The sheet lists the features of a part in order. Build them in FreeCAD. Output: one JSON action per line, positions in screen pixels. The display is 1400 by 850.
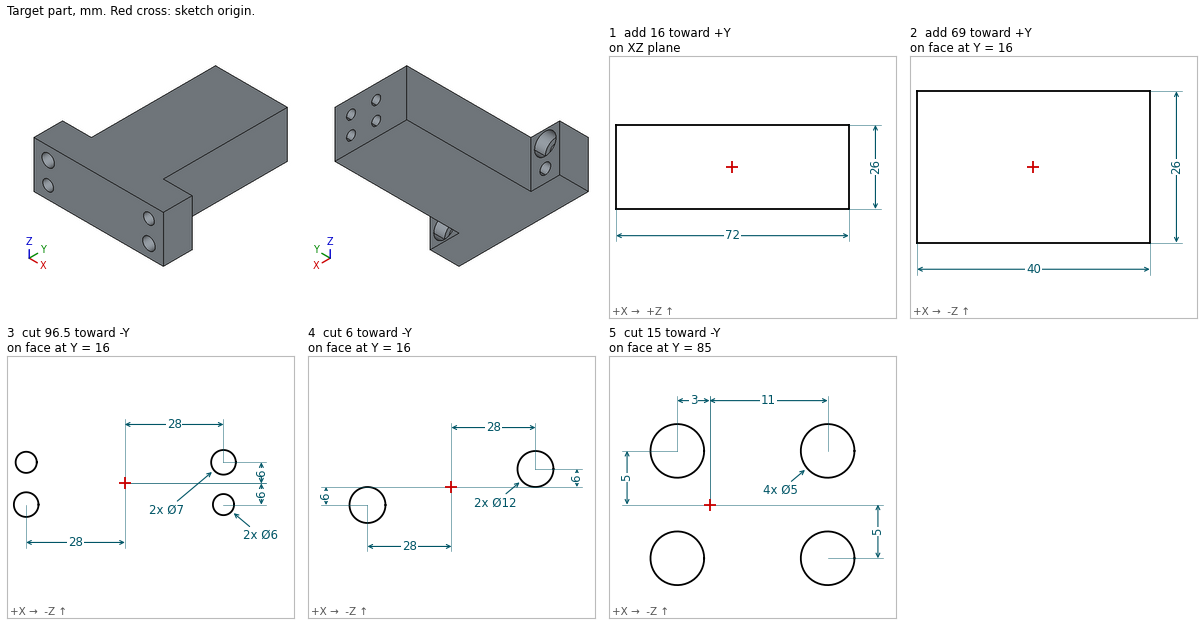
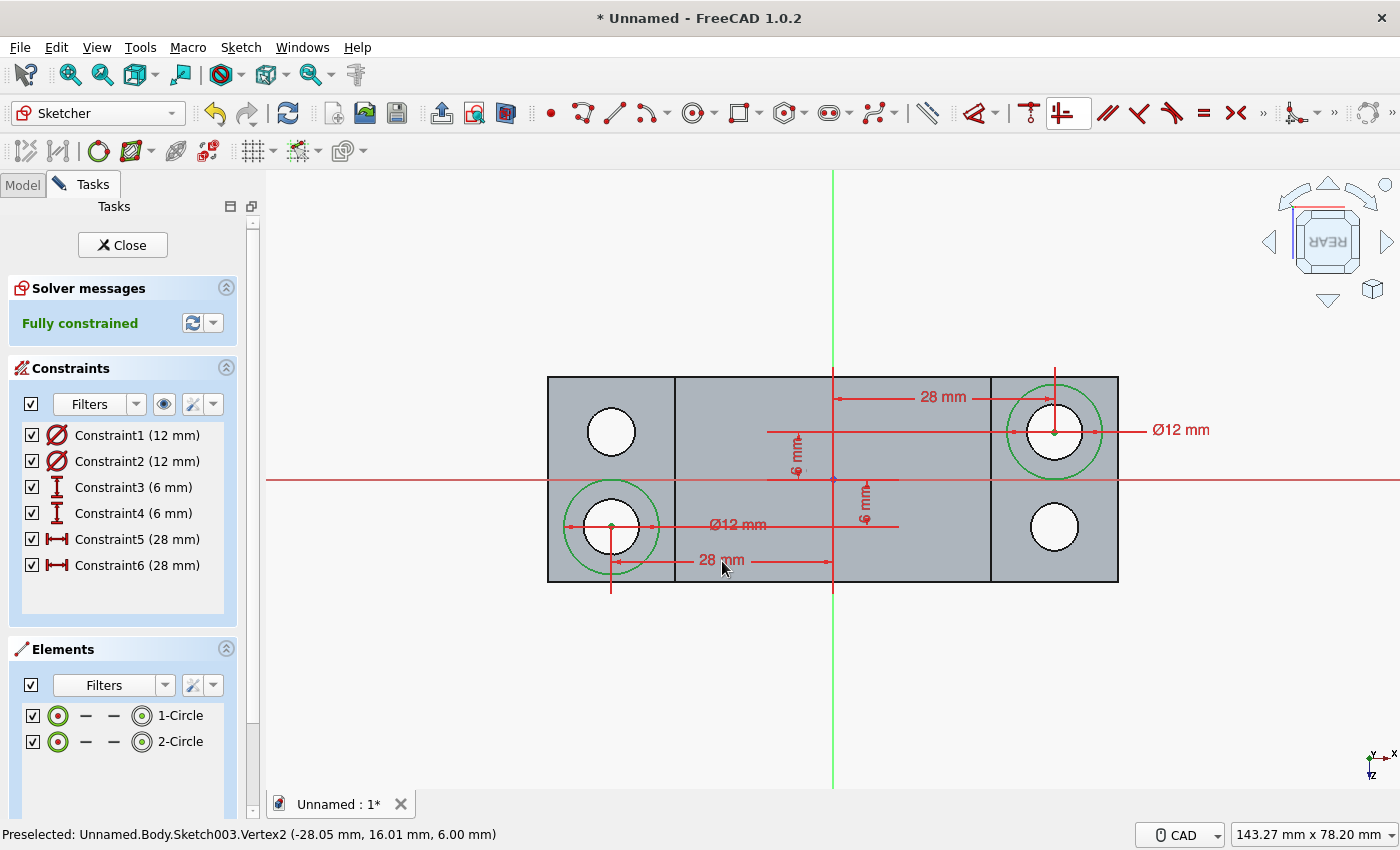
{"action": "left_click", "coordinate": [123, 245]}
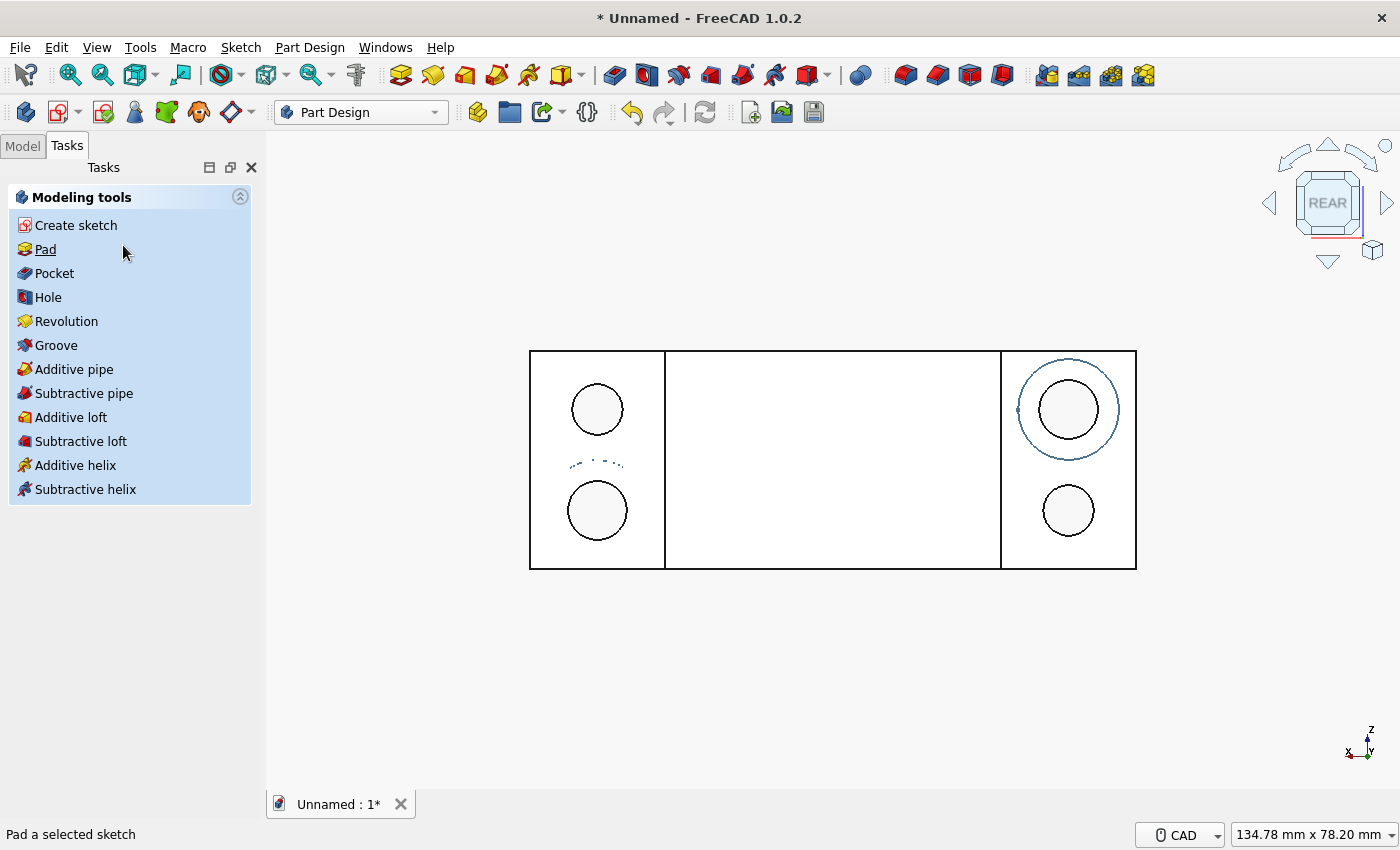
{"action": "left_click", "coordinate": [616, 76]}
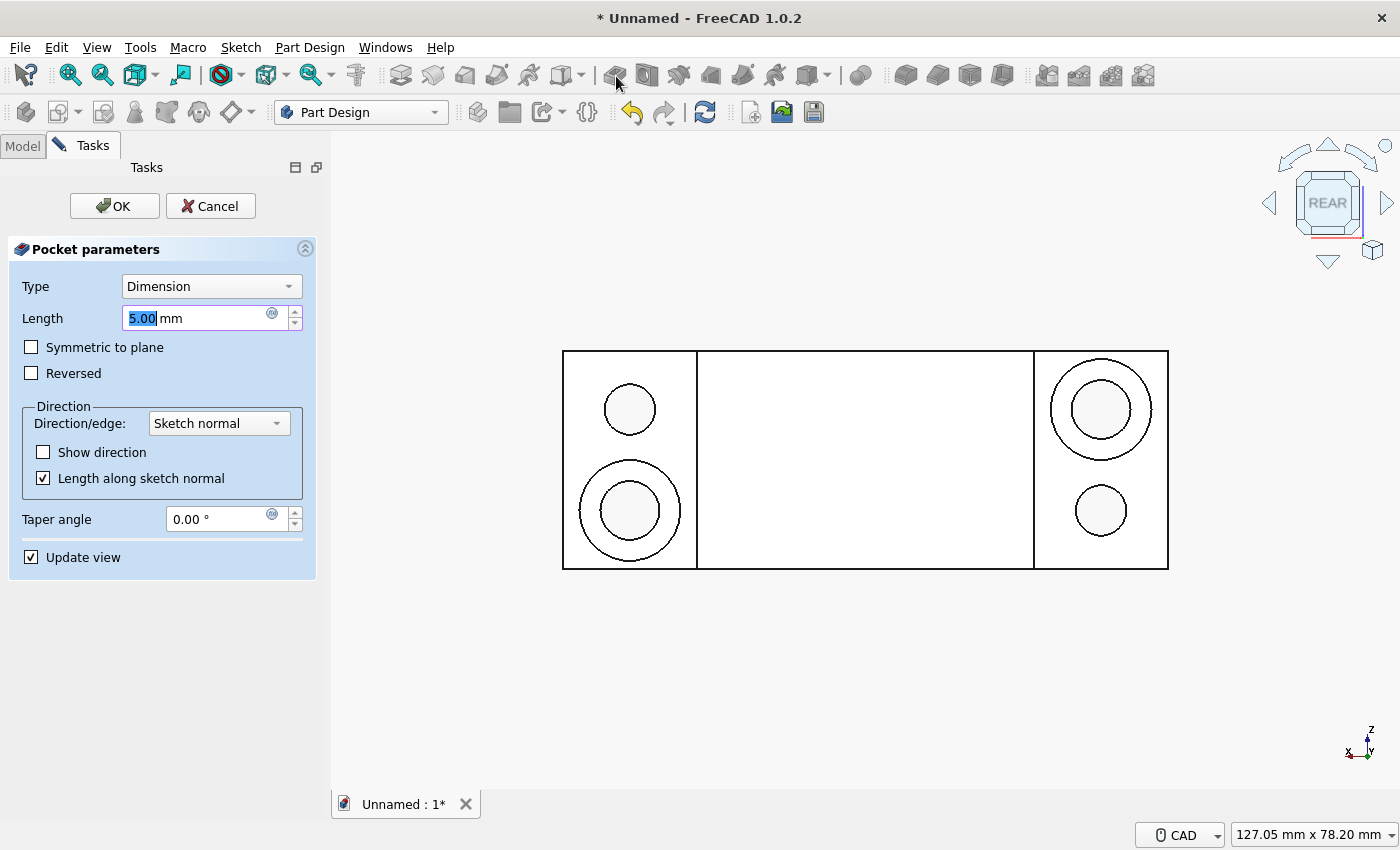
{"action": "type", "text": "6"}
{"action": "key", "text": "Tab"}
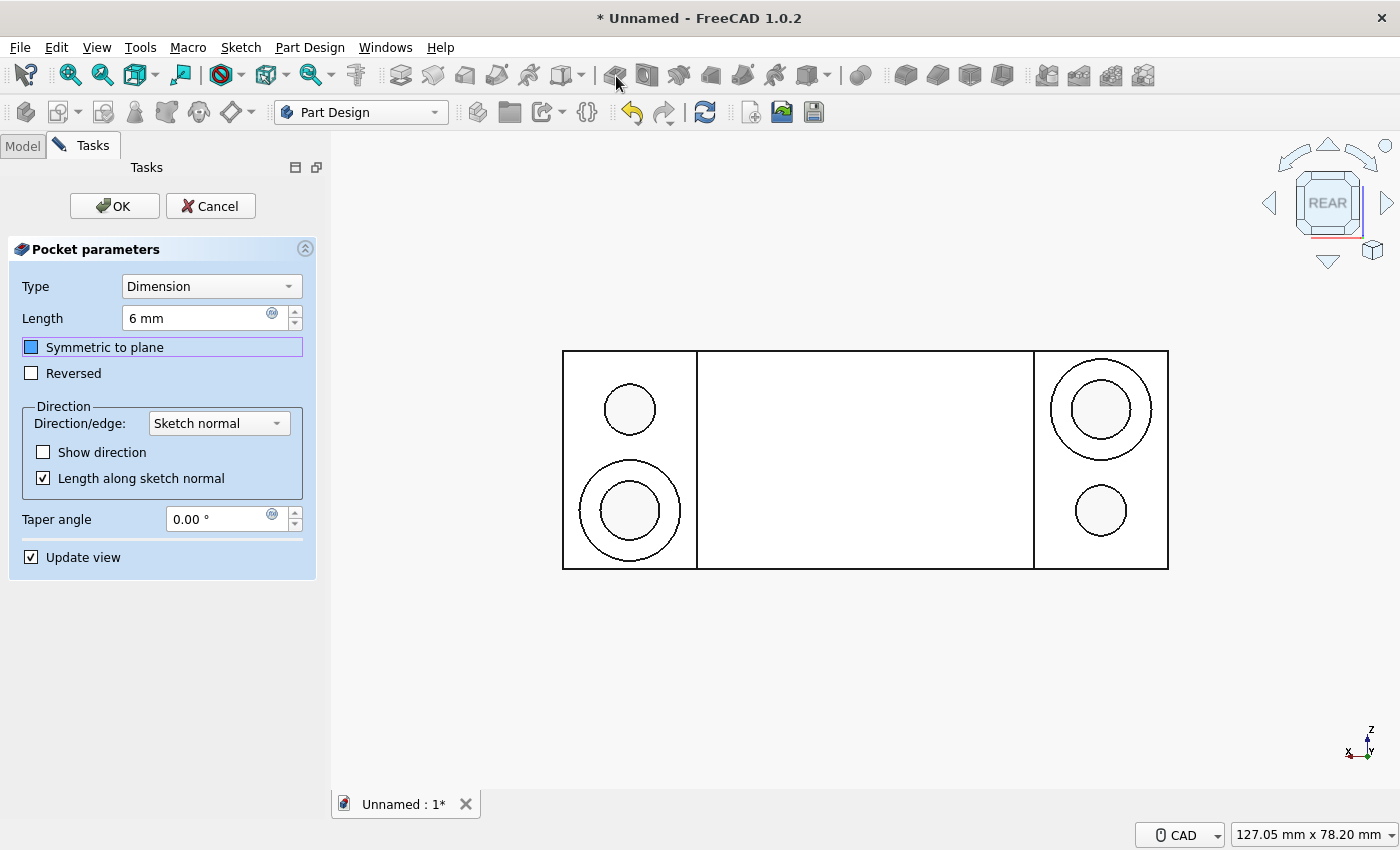
{"action": "left_click", "coordinate": [115, 206]}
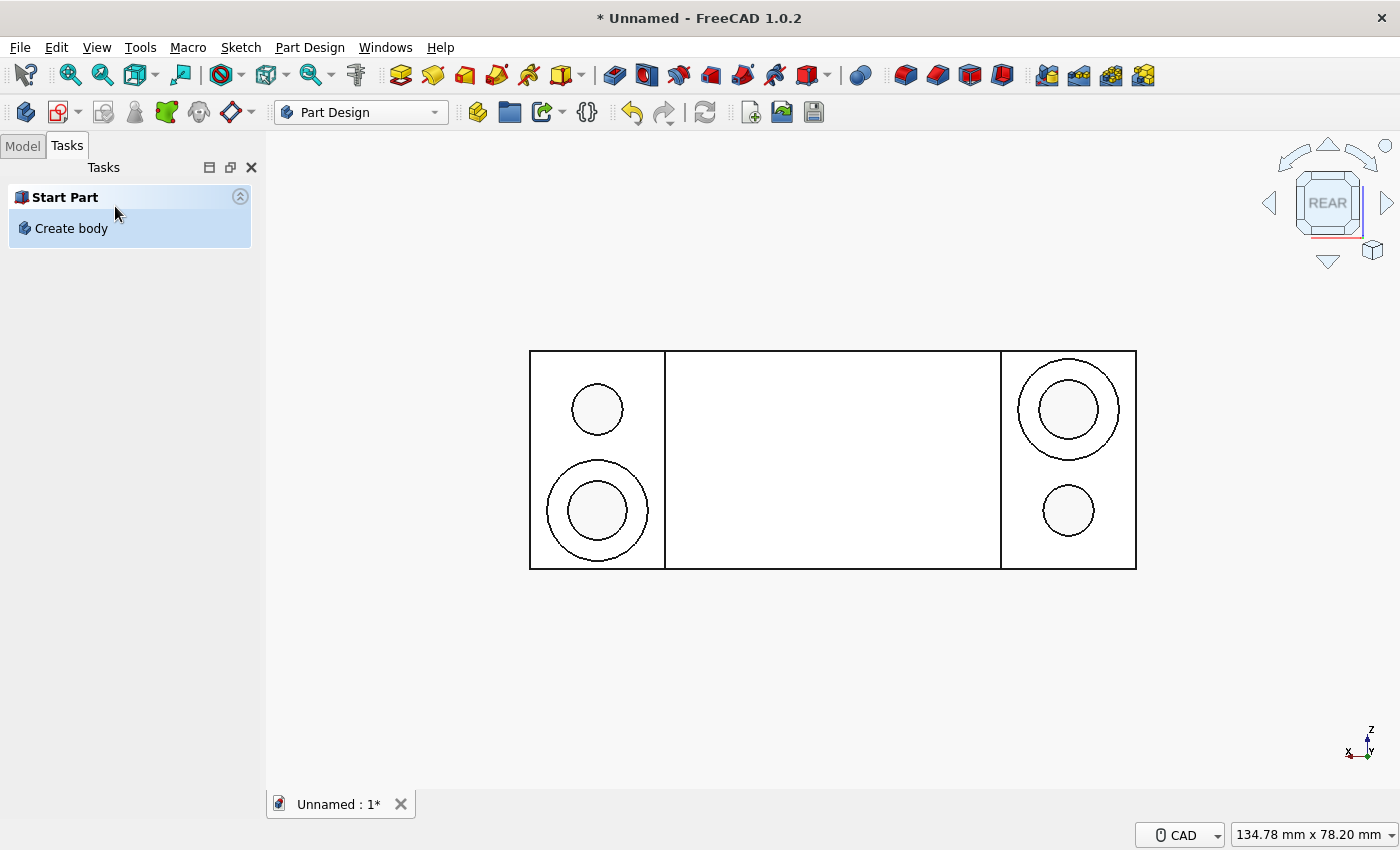
{"action": "left_click", "coordinate": [785, 459]}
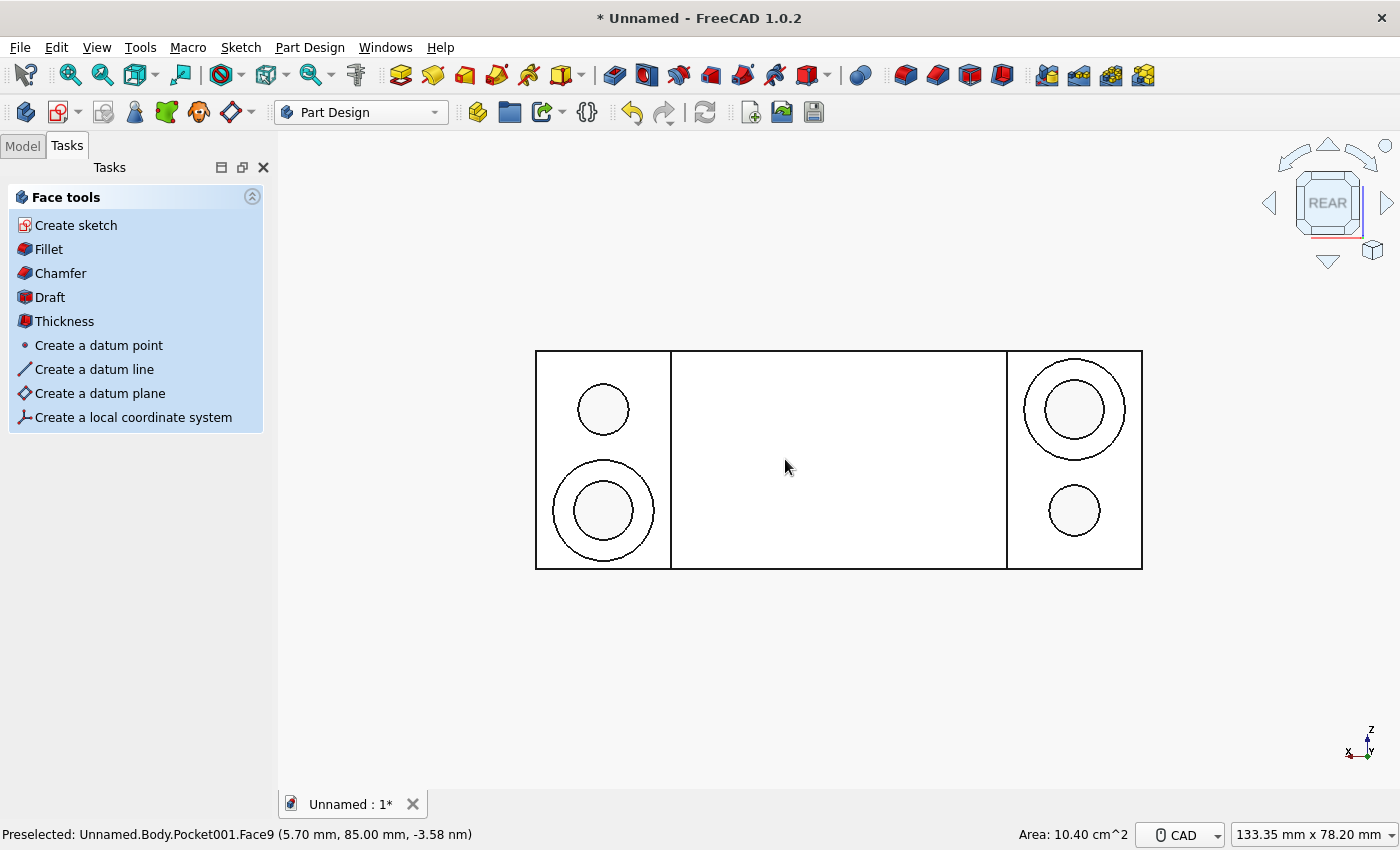
{"action": "left_click", "coordinate": [58, 112]}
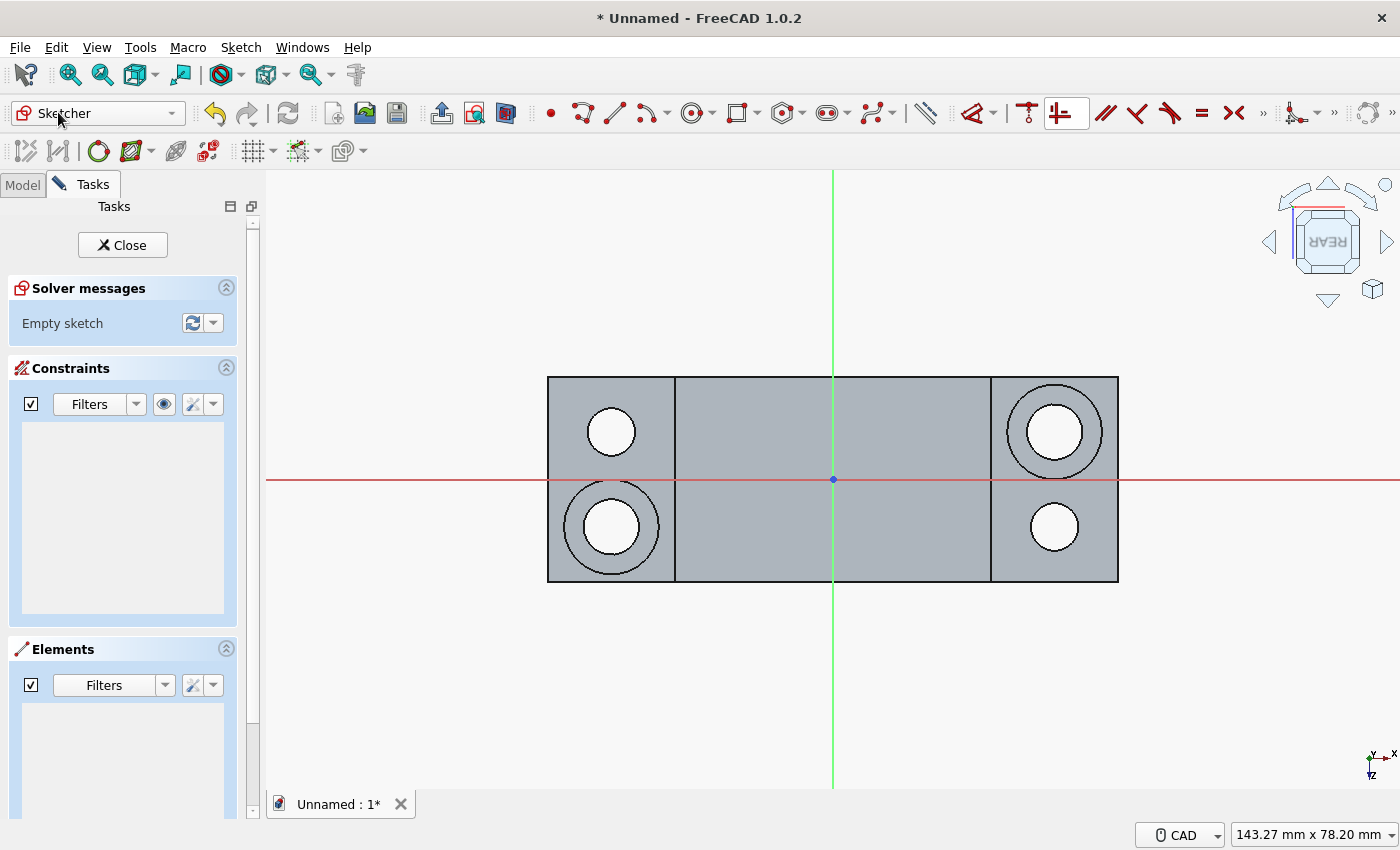
{"action": "scroll", "coordinate": [908, 479], "scroll_direction": "up", "scroll_amount": 6}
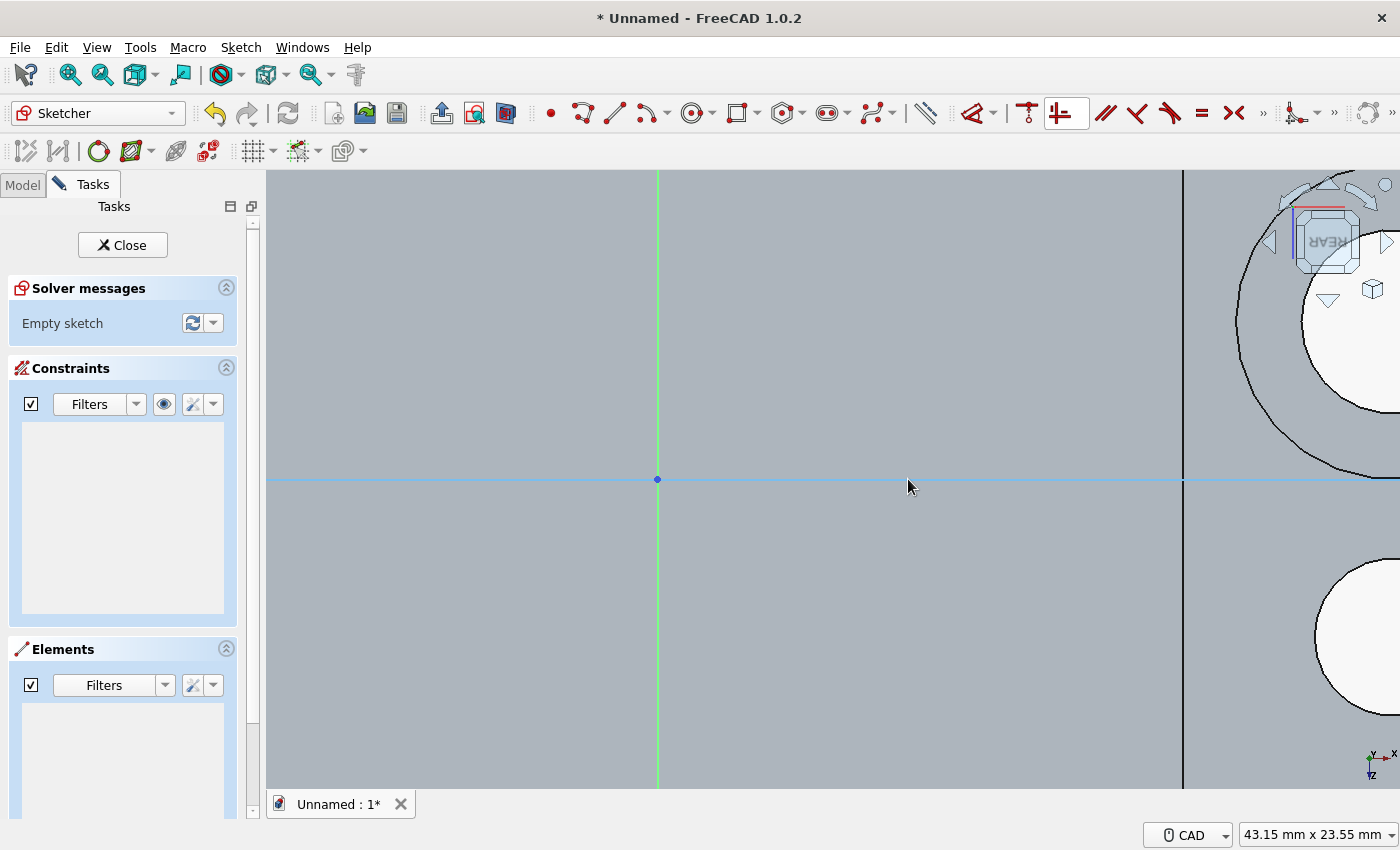
{"action": "key", "text": "g c"}